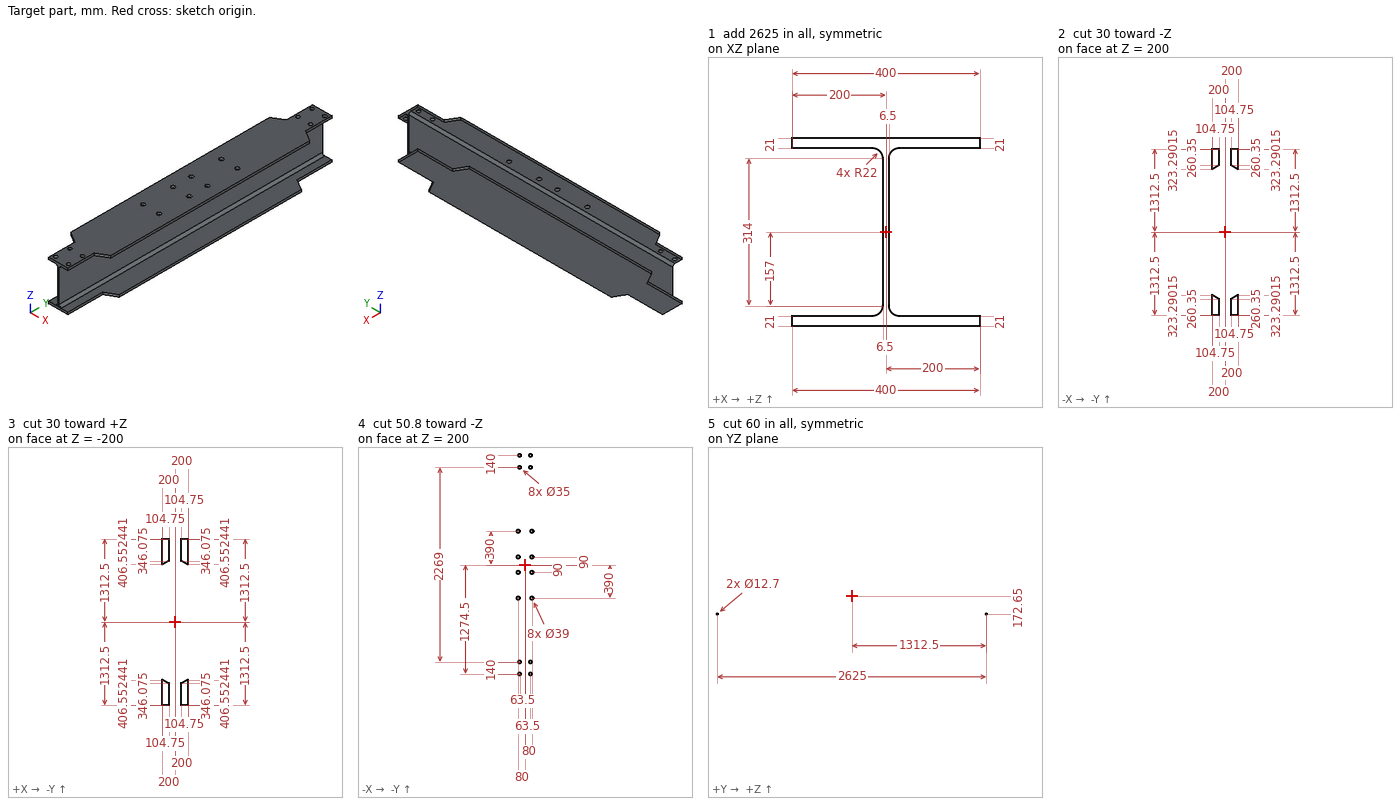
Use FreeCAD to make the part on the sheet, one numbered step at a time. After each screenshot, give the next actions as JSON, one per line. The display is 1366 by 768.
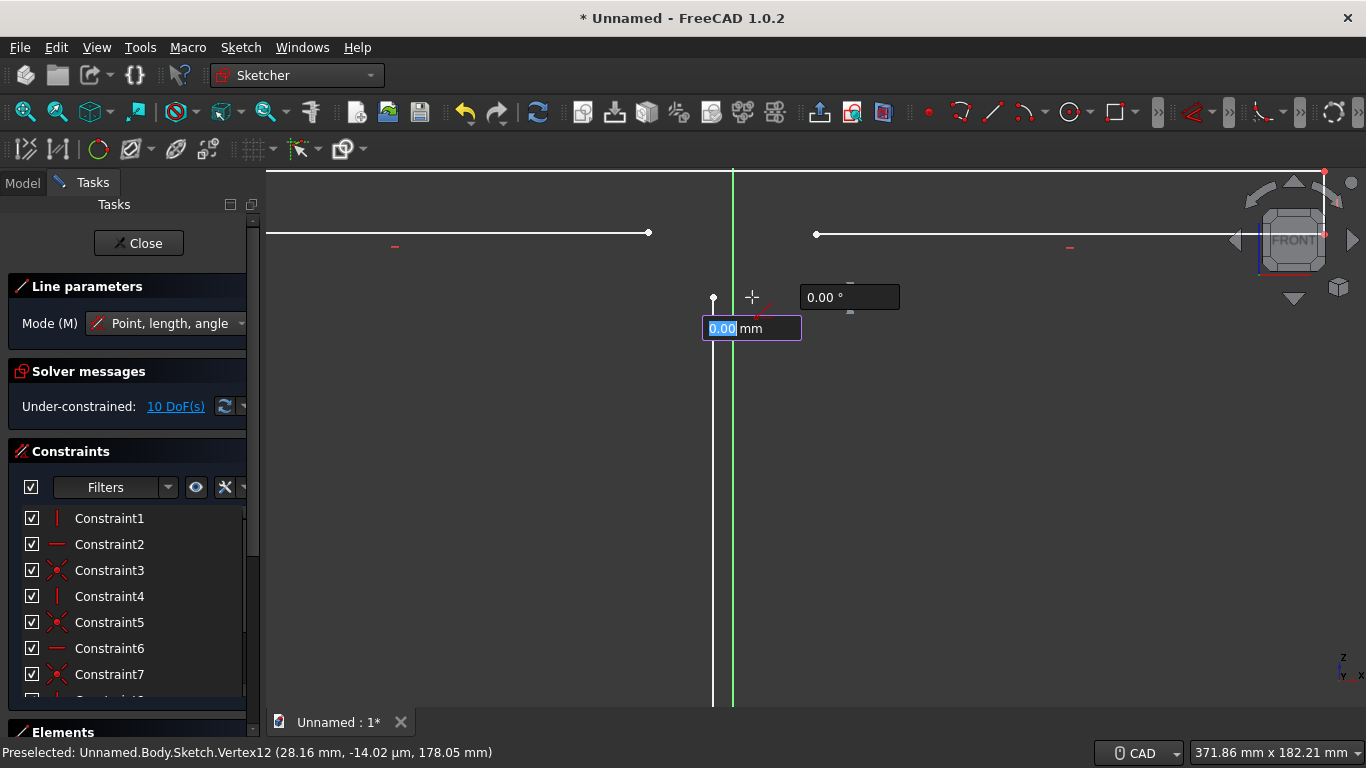
{"action": "scroll", "coordinate": [754, 298], "scroll_direction": "down", "scroll_amount": 6}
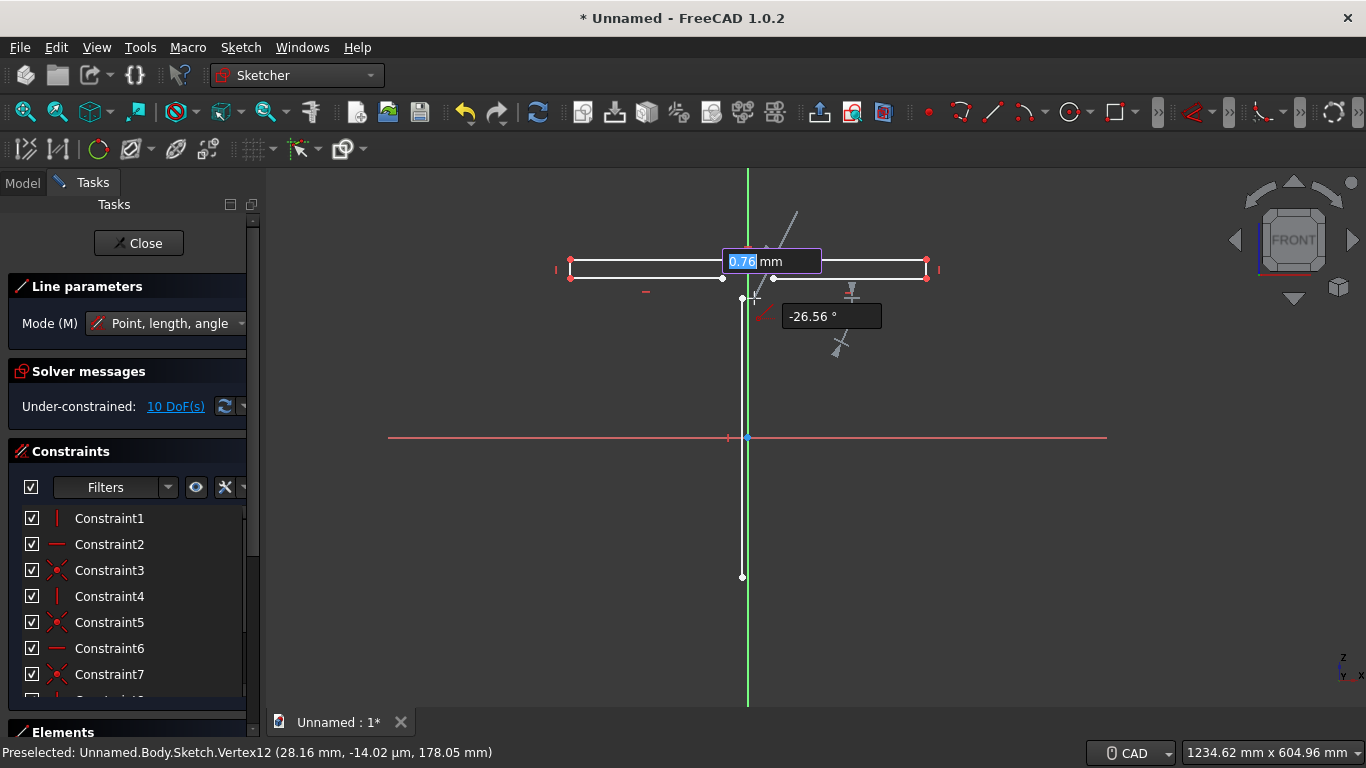
{"action": "scroll", "coordinate": [754, 578], "scroll_direction": "up", "scroll_amount": 6}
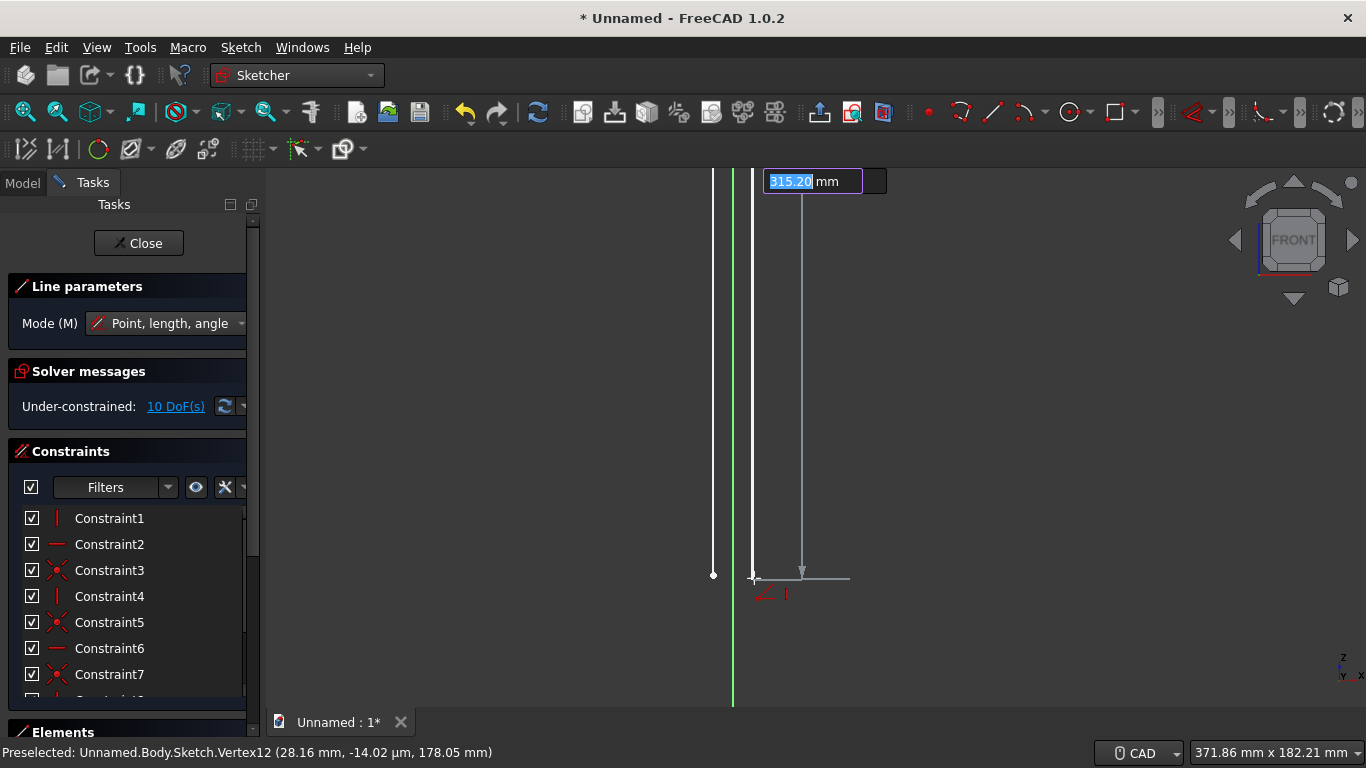
{"action": "left_click", "coordinate": [752, 575]}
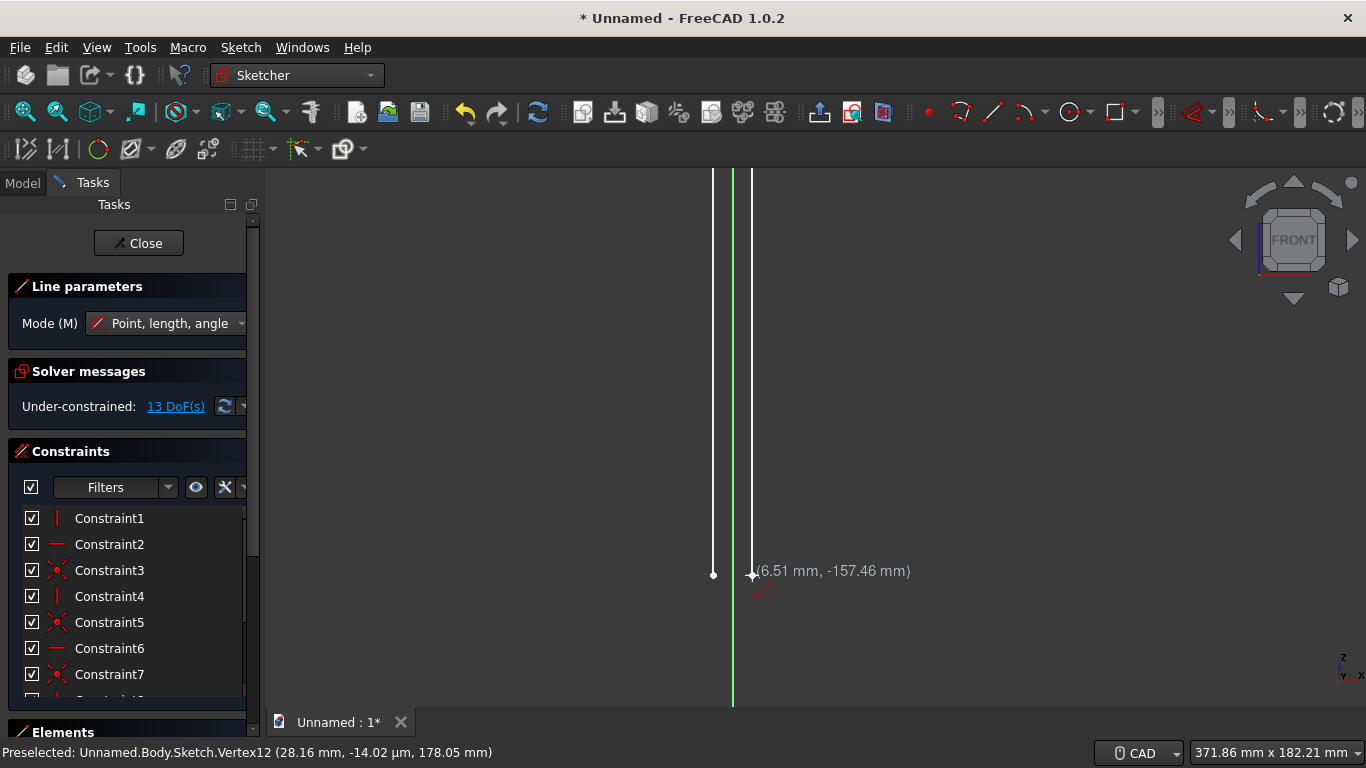
{"action": "left_click", "coordinate": [962, 112]}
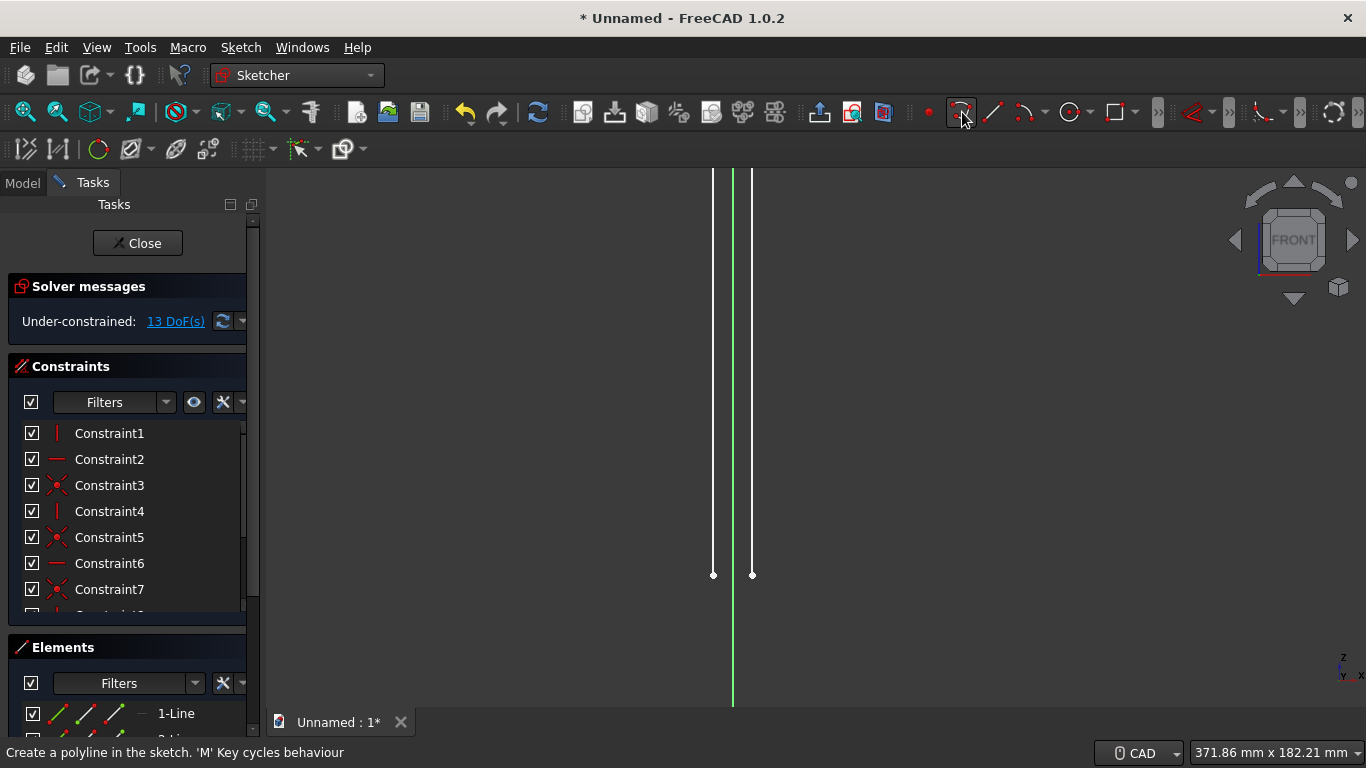
{"action": "left_click", "coordinate": [817, 640]}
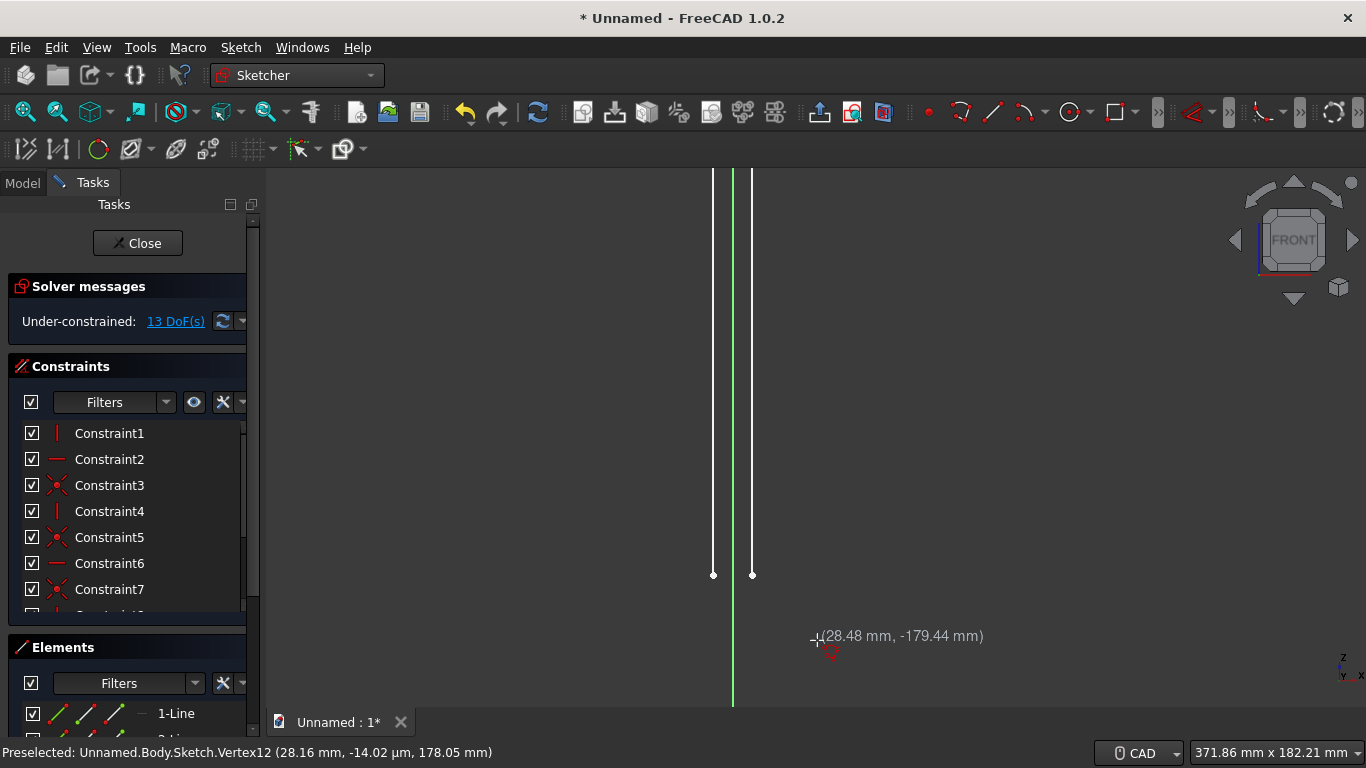
{"action": "scroll", "coordinate": [754, 579], "scroll_direction": "down", "scroll_amount": 6}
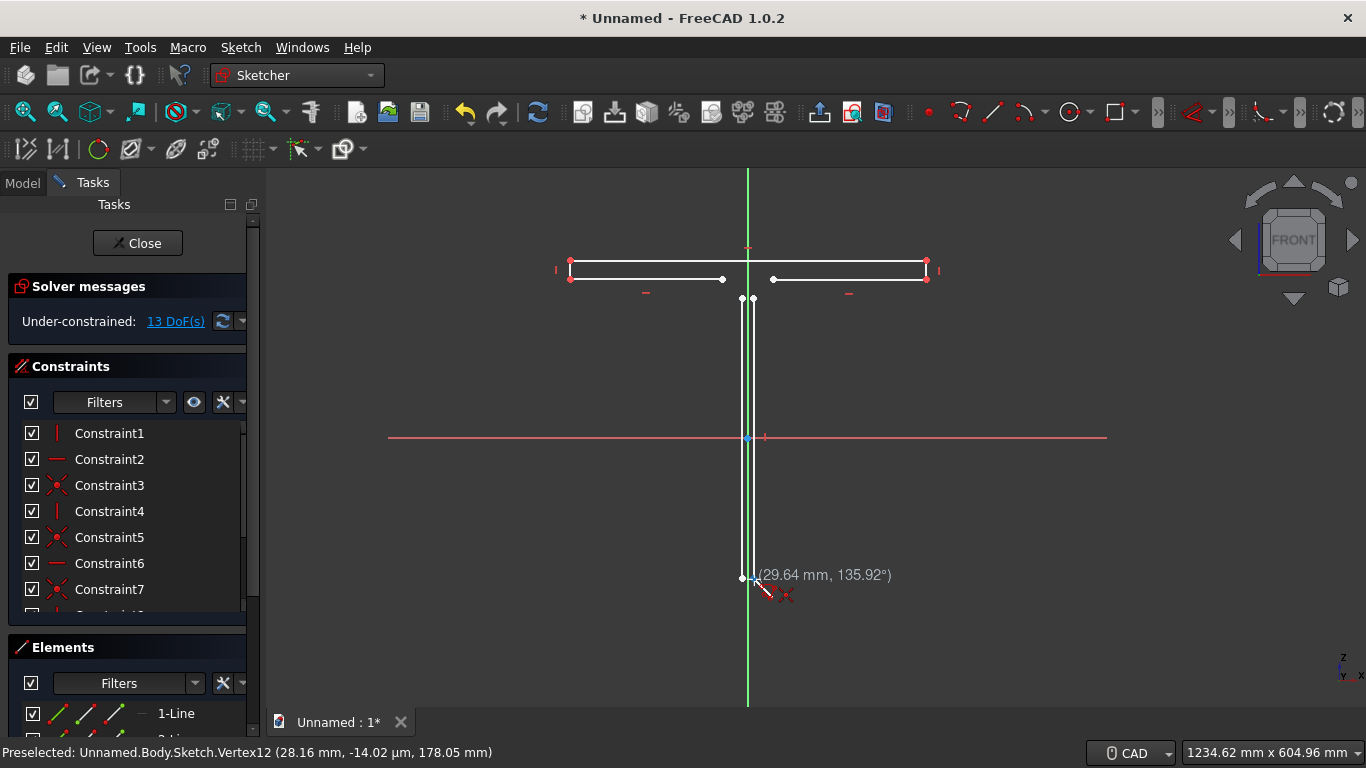
{"action": "left_click", "coordinate": [926, 598]}
{"action": "left_click", "coordinate": [926, 617]}
{"action": "left_click", "coordinate": [570, 617]}
{"action": "left_click", "coordinate": [570, 598]}
{"action": "left_click", "coordinate": [723, 598]}
{"action": "right_click", "coordinate": [723, 598]}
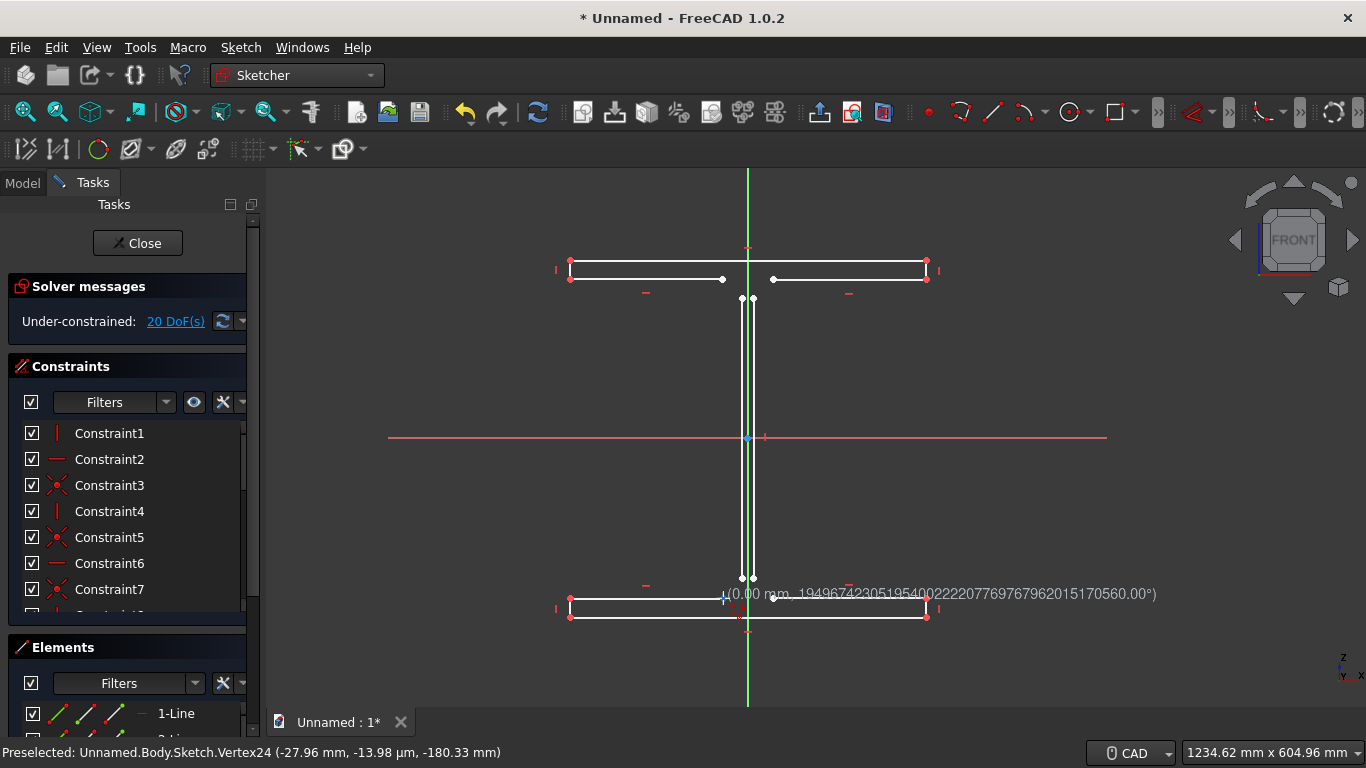
{"action": "left_click", "coordinate": [1048, 112]}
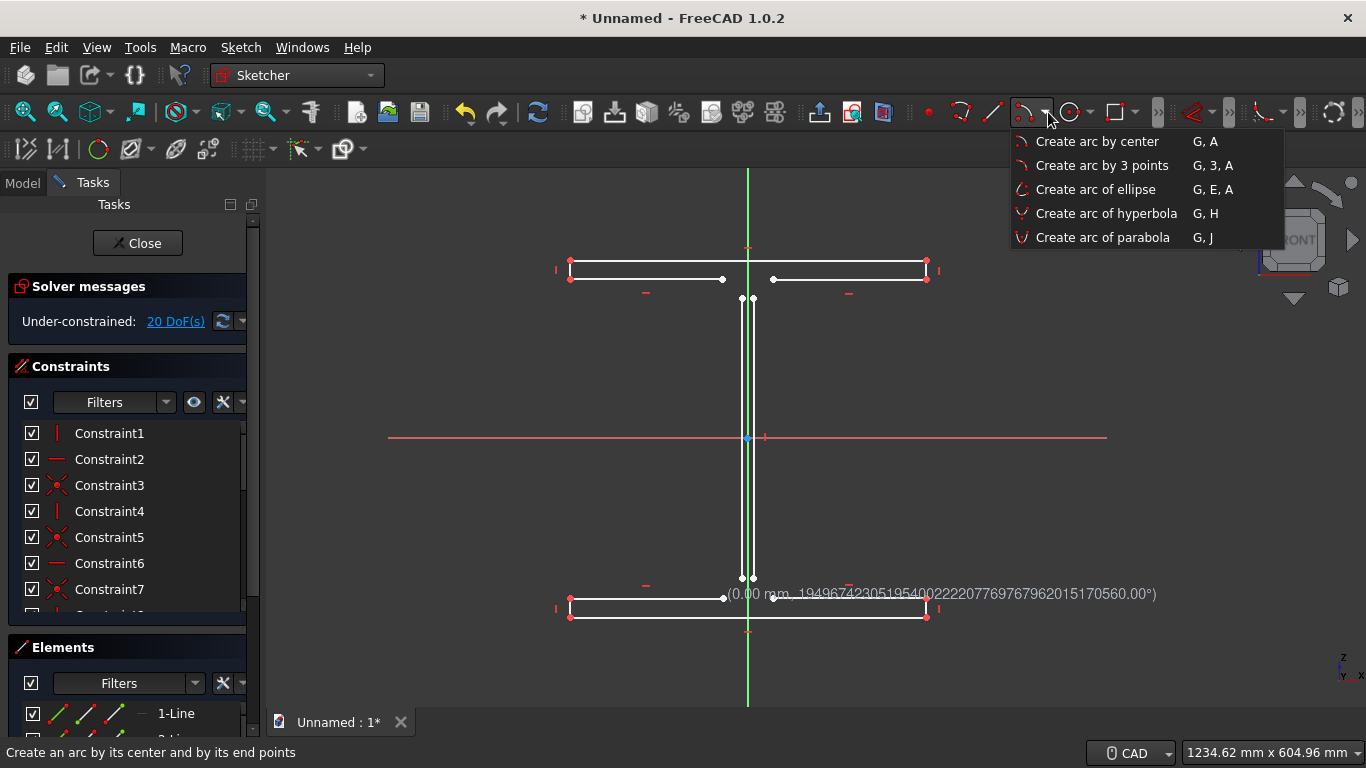
{"action": "left_click", "coordinate": [1148, 165]}